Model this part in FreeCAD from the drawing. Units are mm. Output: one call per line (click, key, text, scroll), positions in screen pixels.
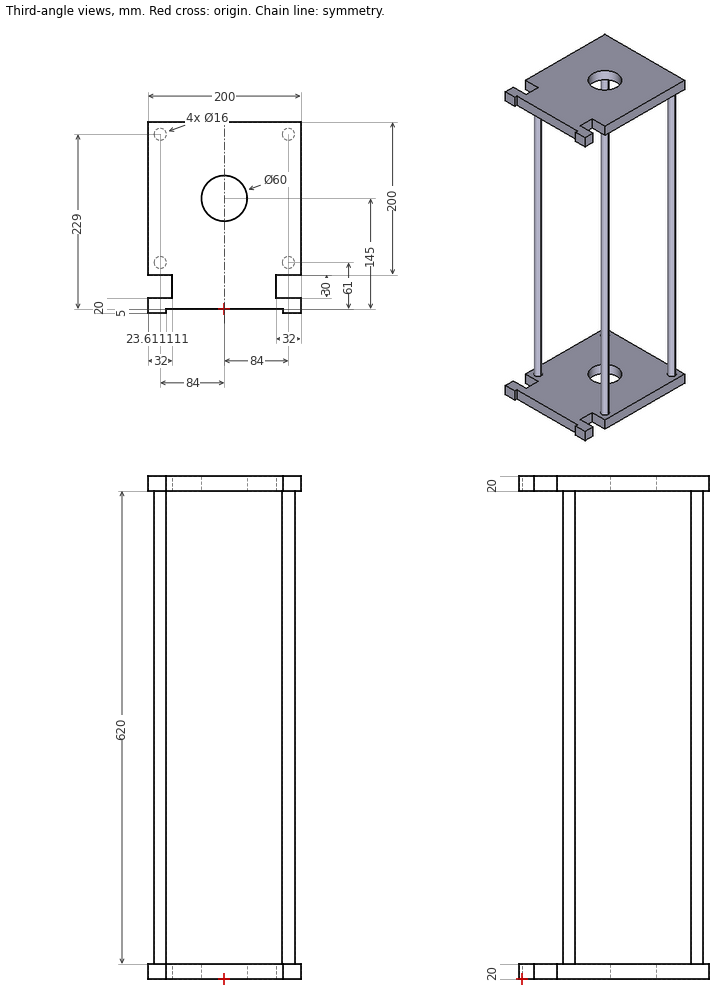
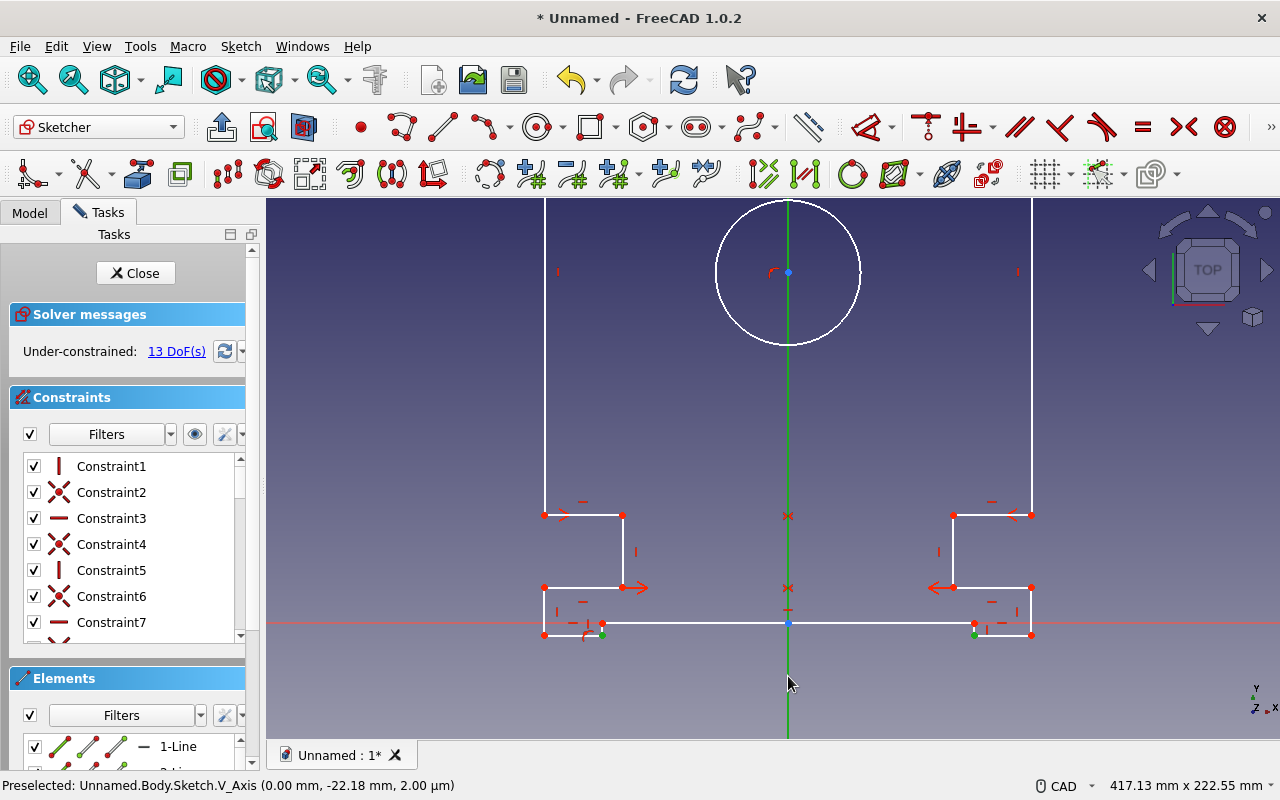
click(1184, 128)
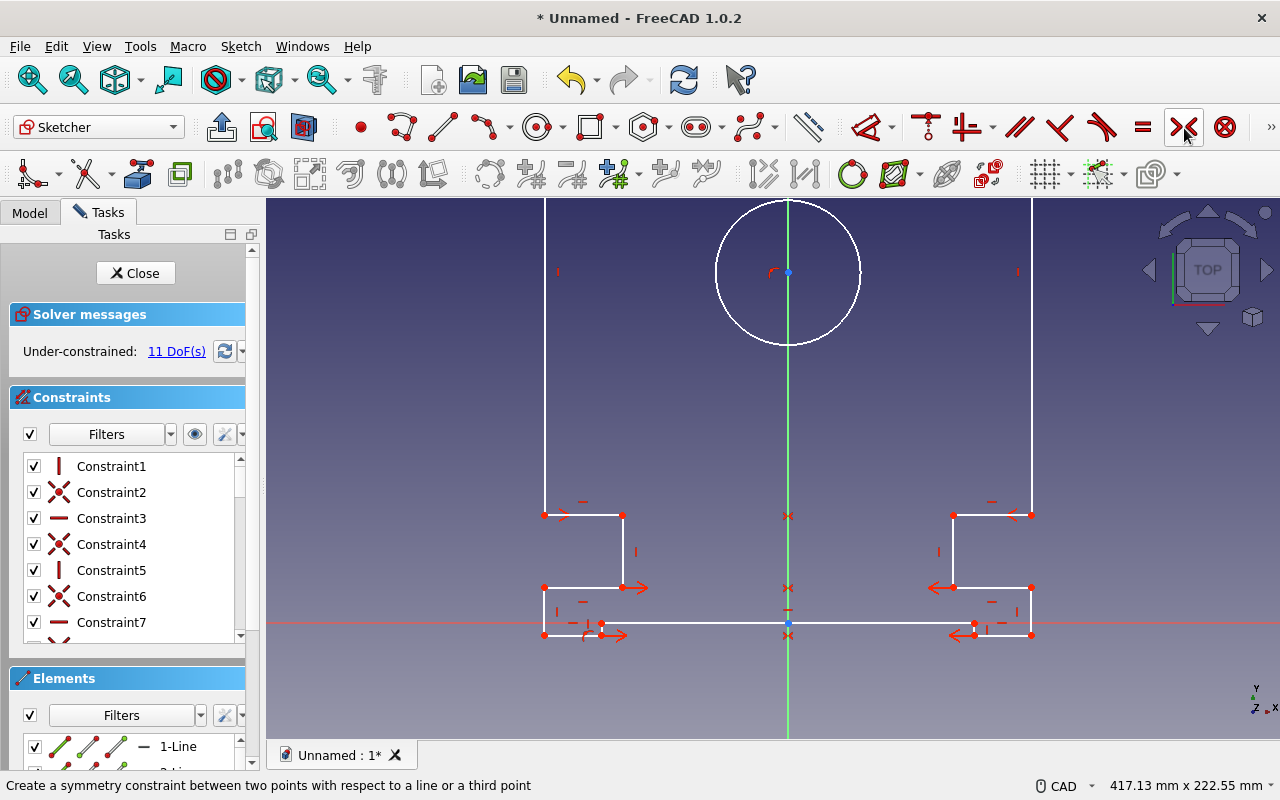
click(866, 128)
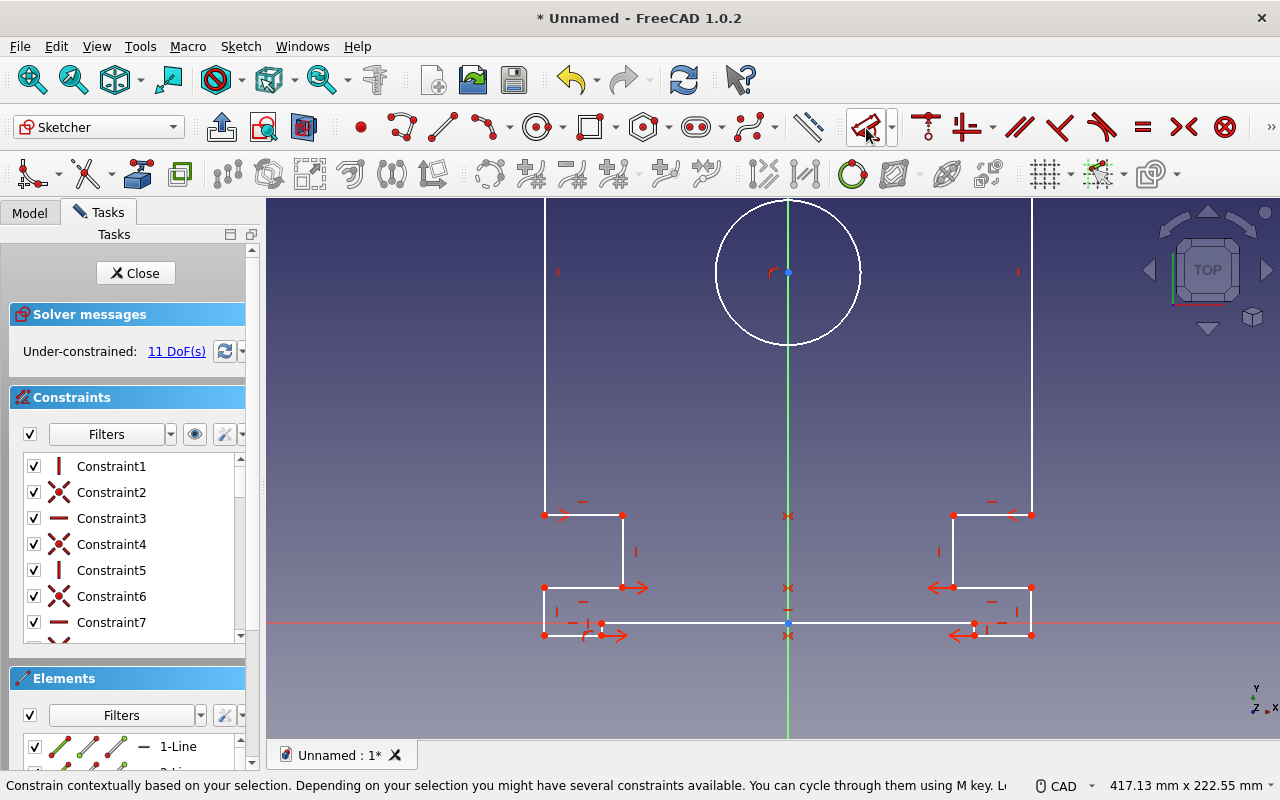
click(737, 324)
click(714, 347)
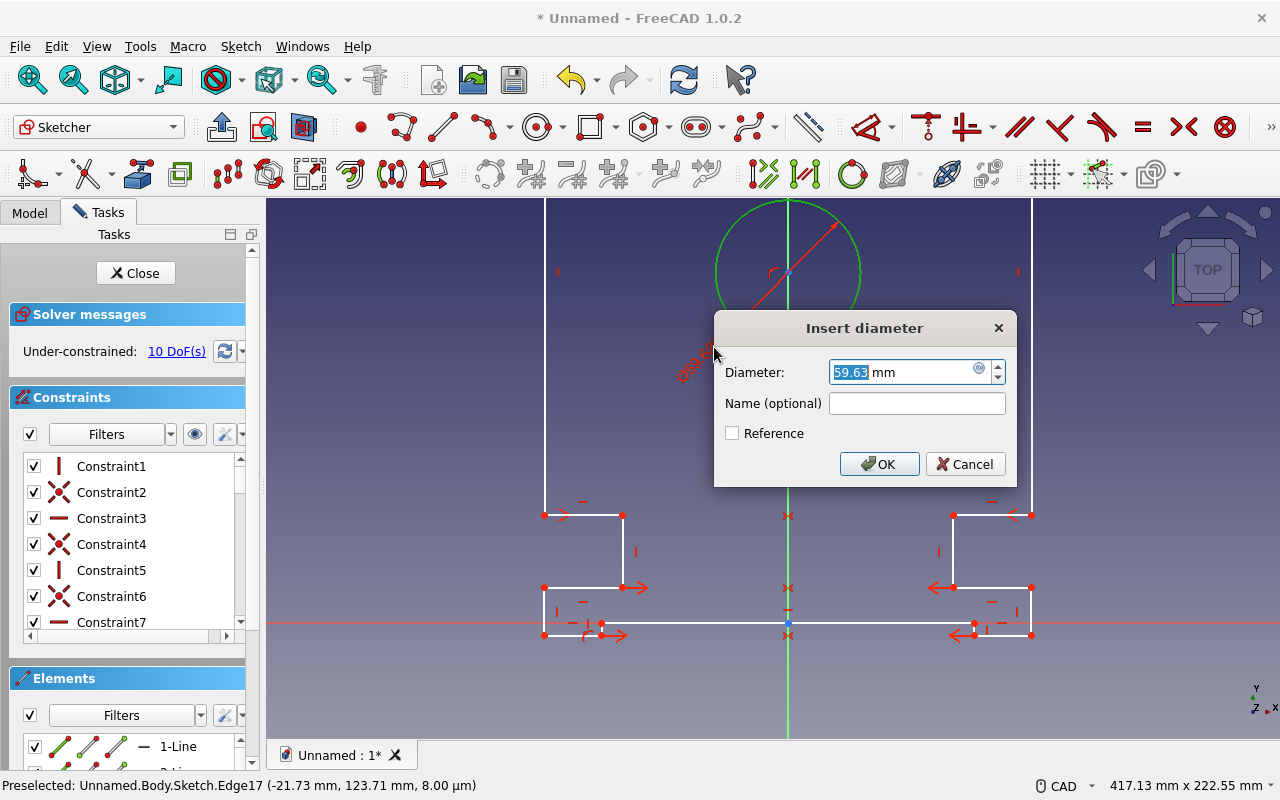
text(60)
key(Return)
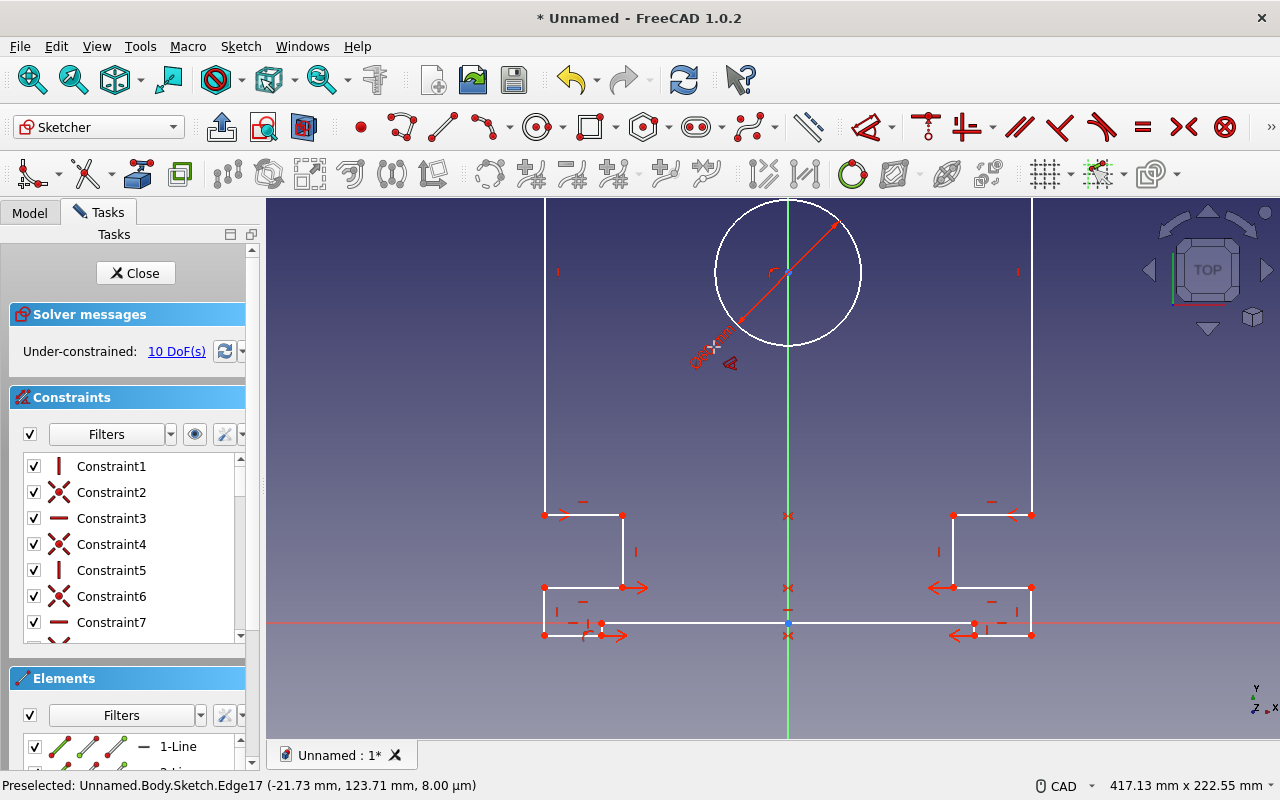
scroll(602, 629, up, 6)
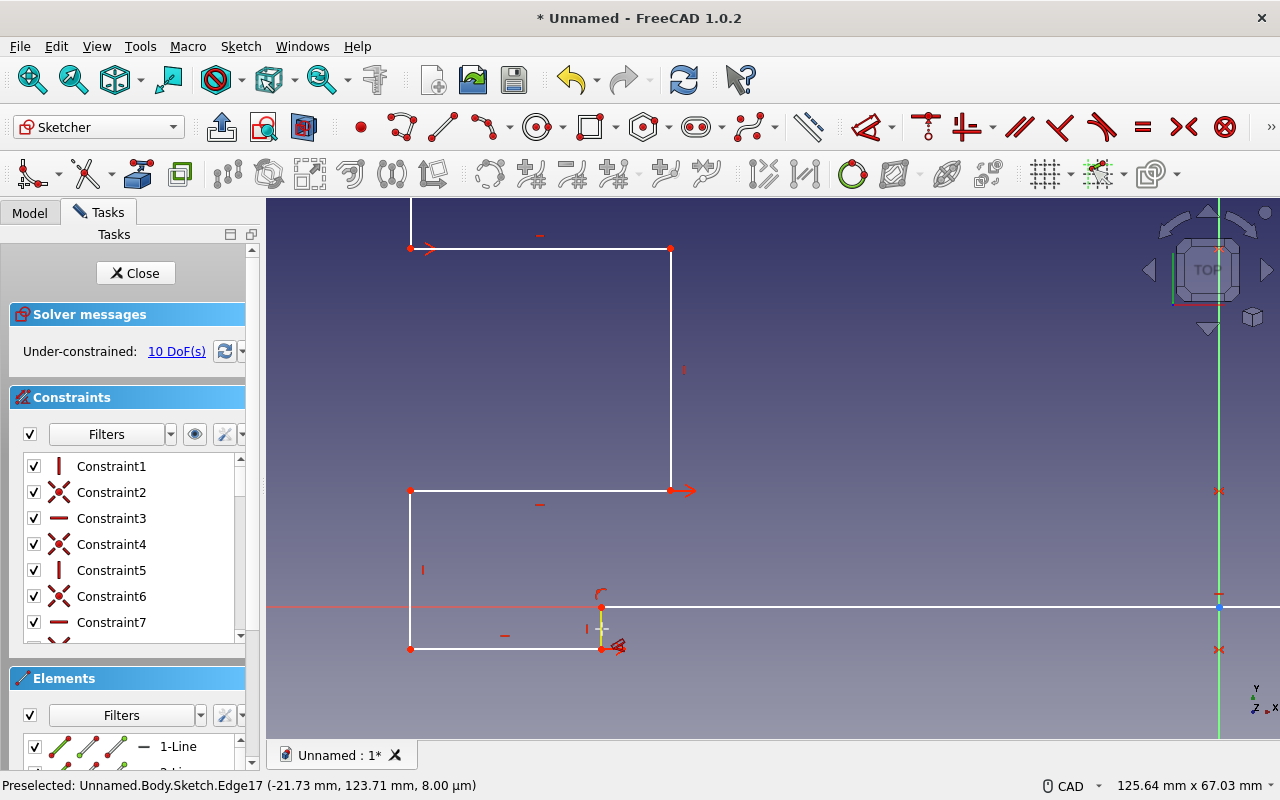
click(601, 628)
click(567, 628)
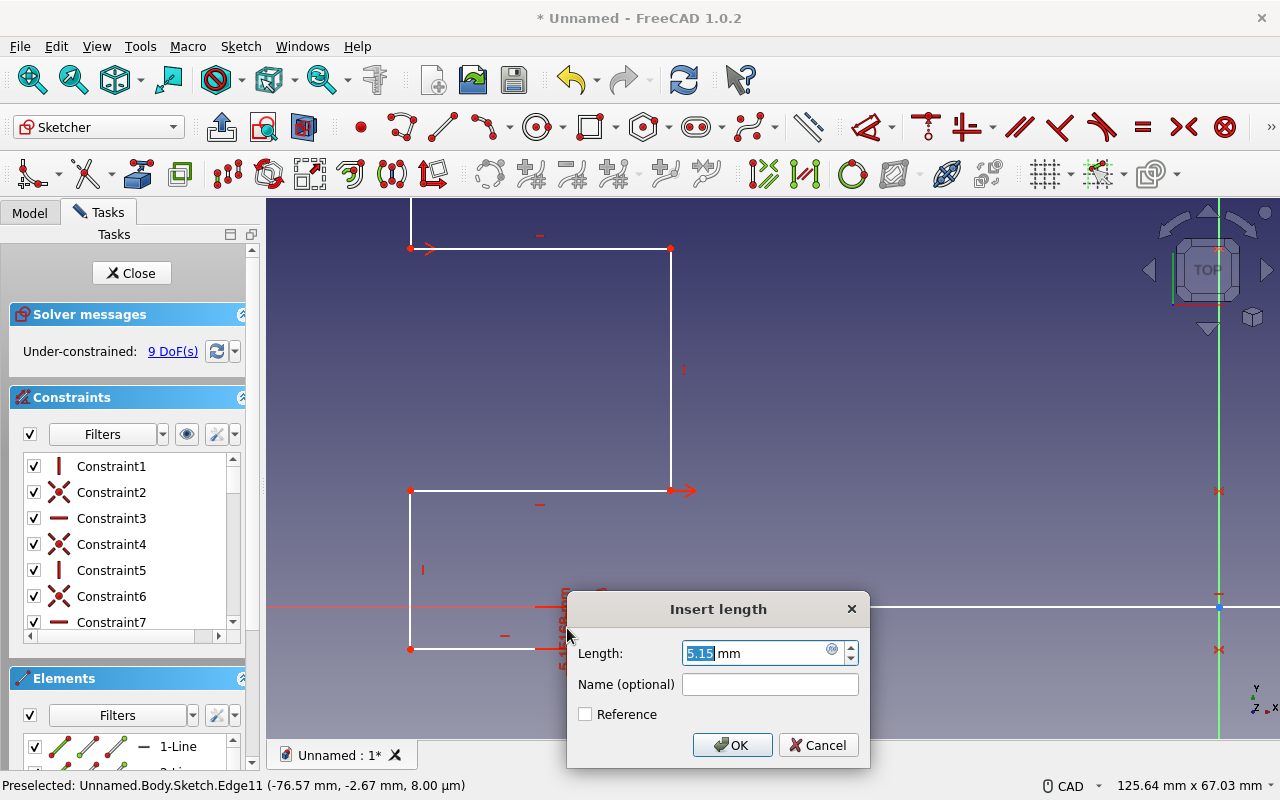
text(5)
key(Return)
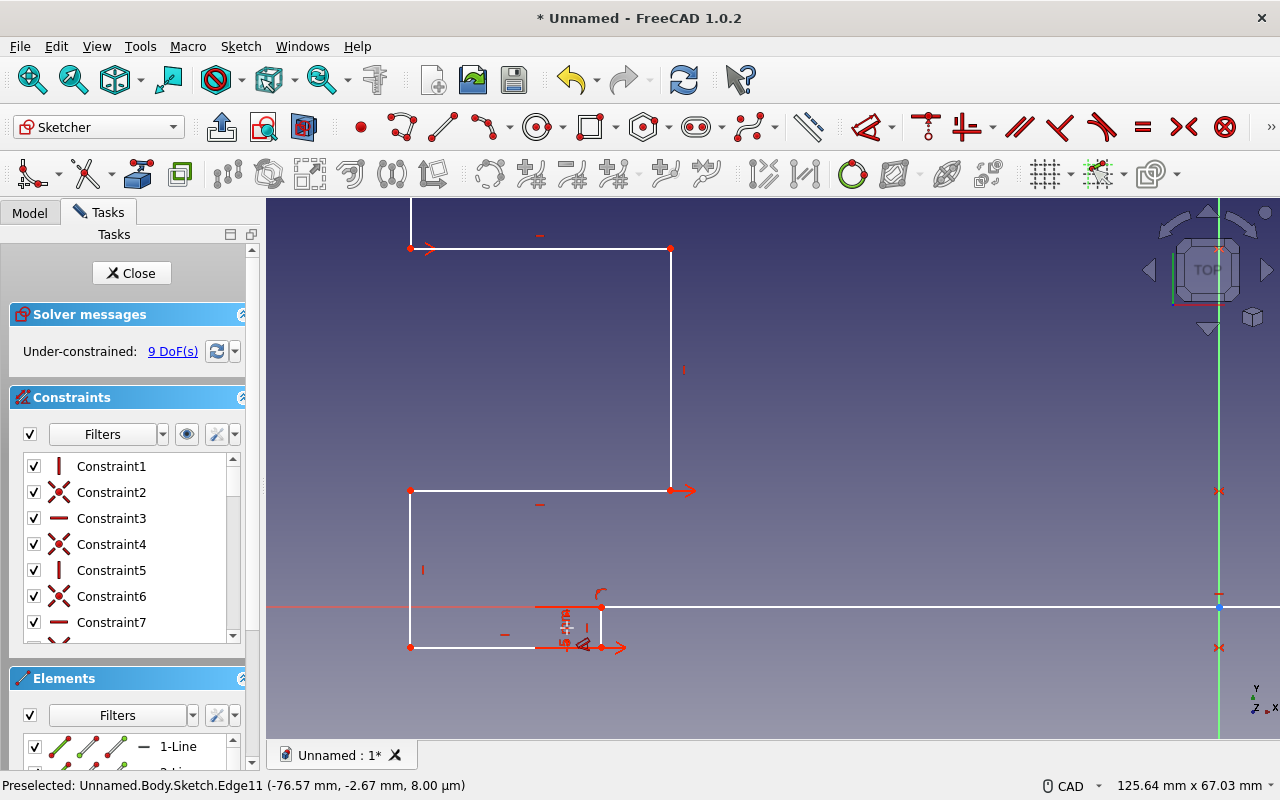
scroll(603, 633, down, 9)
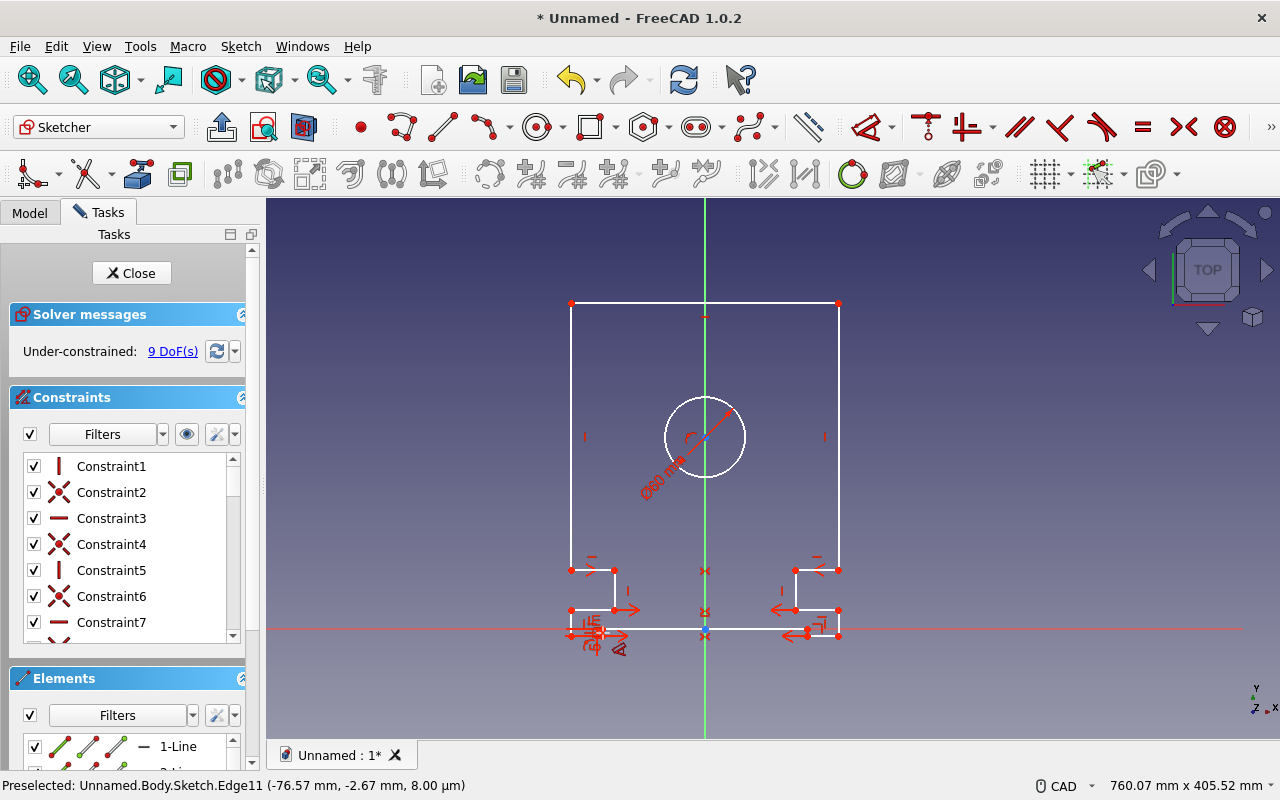
click(796, 598)
click(830, 590)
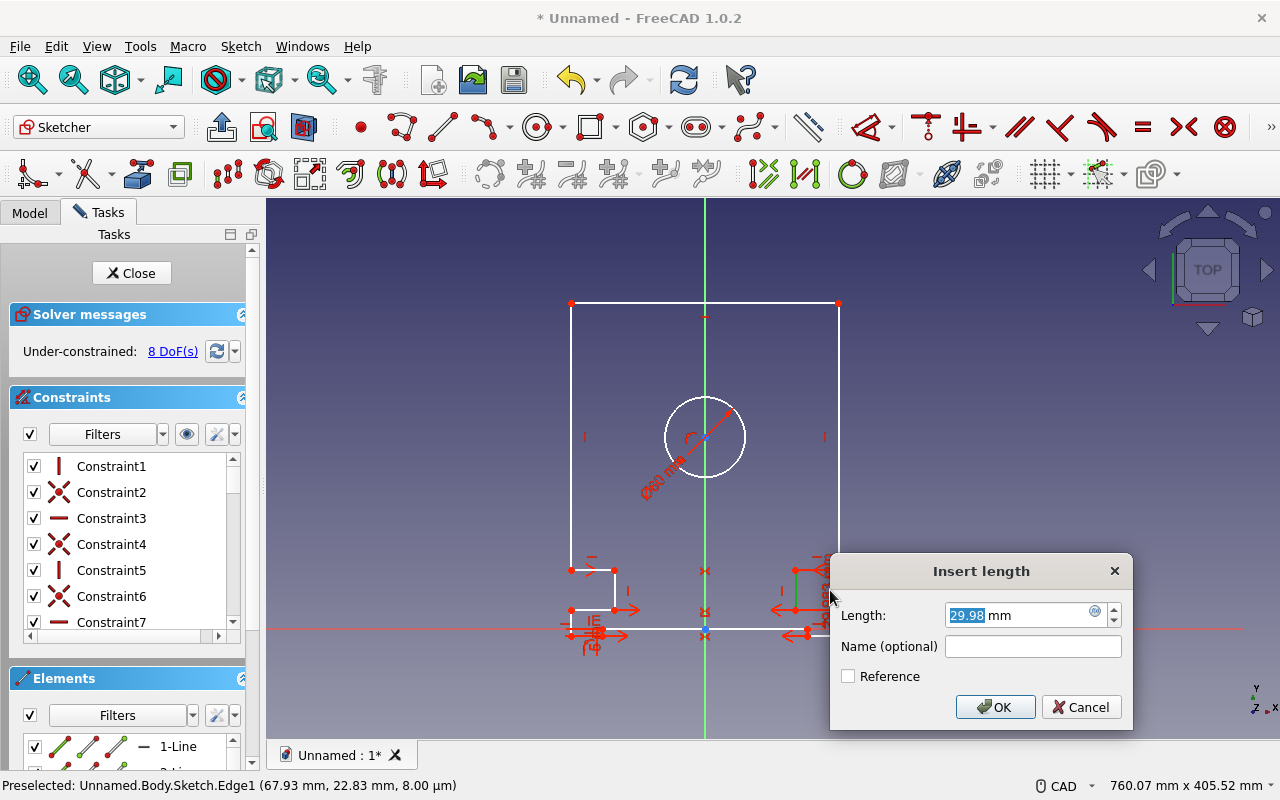
text(30)
key(Return)